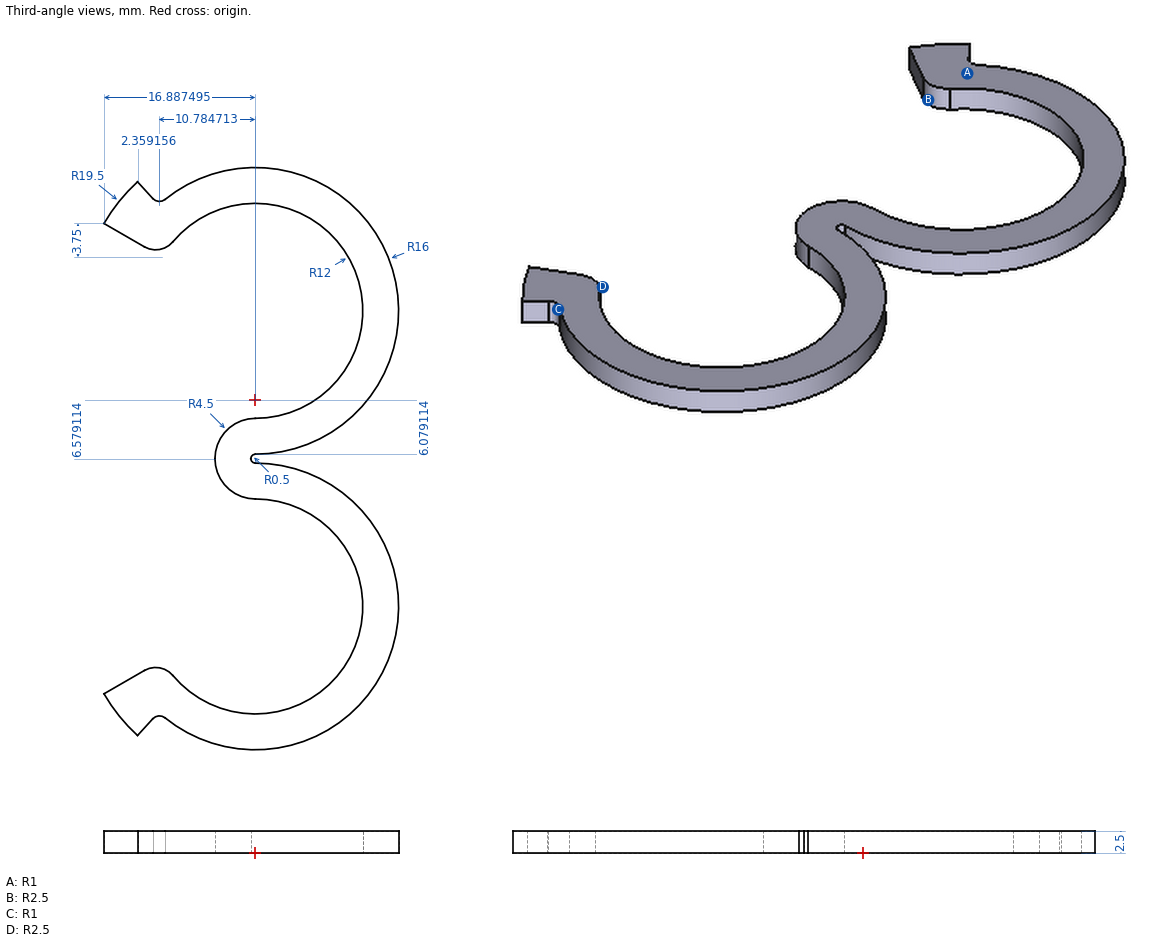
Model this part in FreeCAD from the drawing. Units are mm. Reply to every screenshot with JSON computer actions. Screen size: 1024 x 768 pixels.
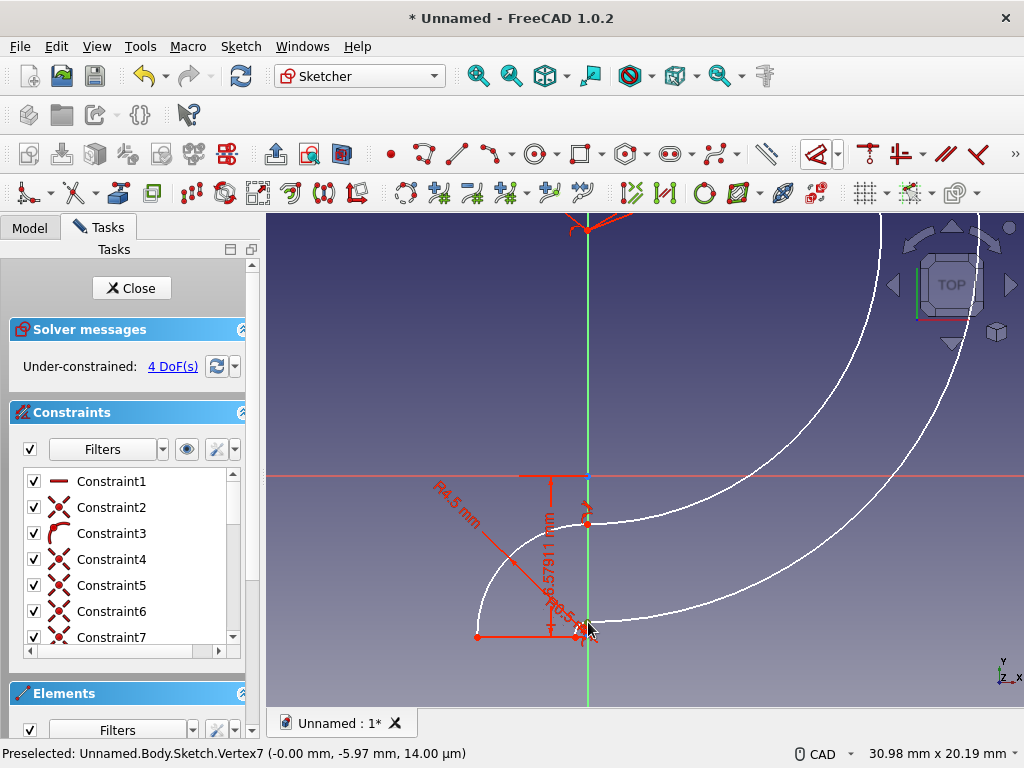
{"action": "left_click", "coordinate": [838, 154]}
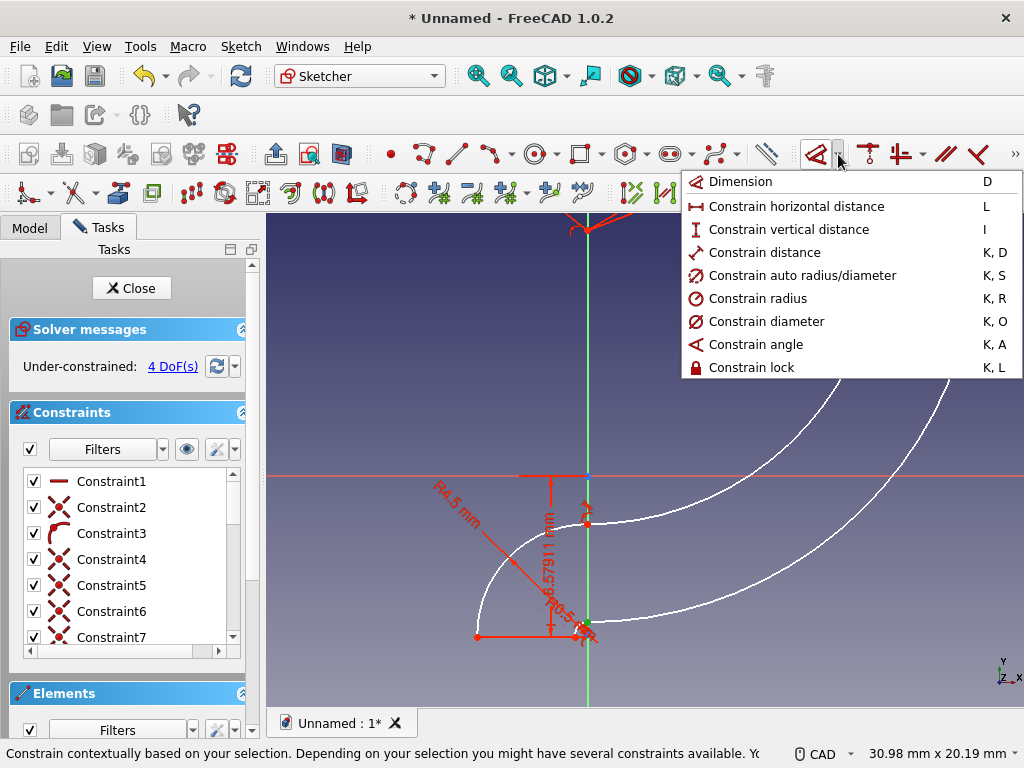
{"action": "left_click", "coordinate": [852, 230]}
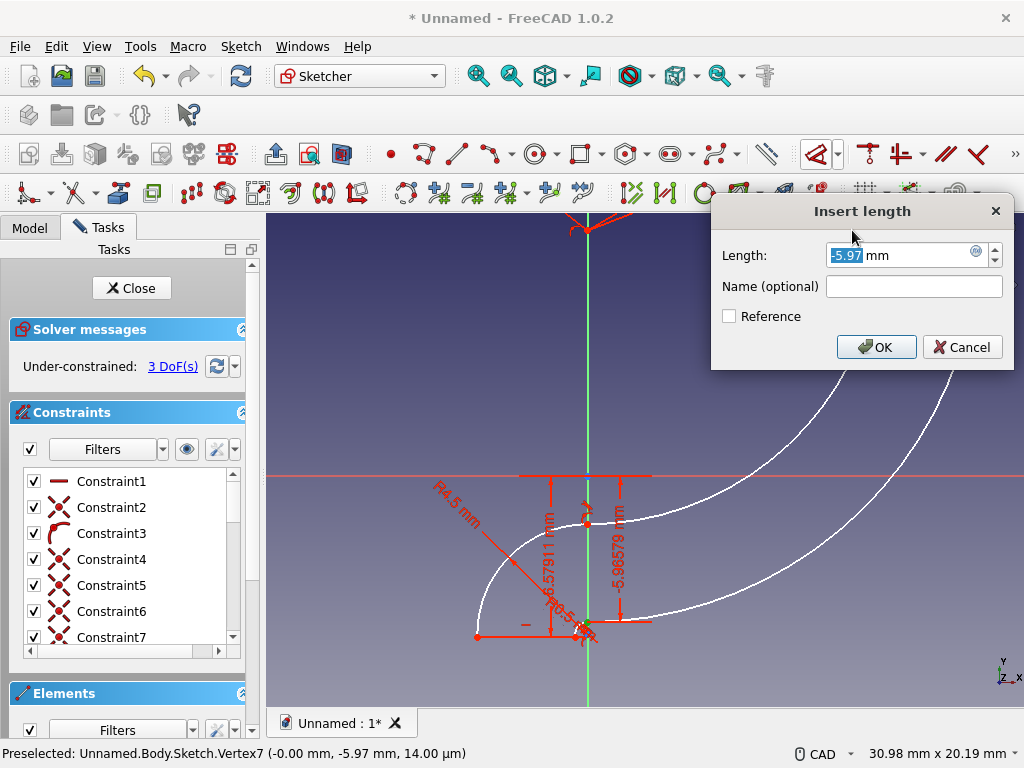
{"action": "type", "text": "-6.079114"}
{"action": "key", "text": "Return"}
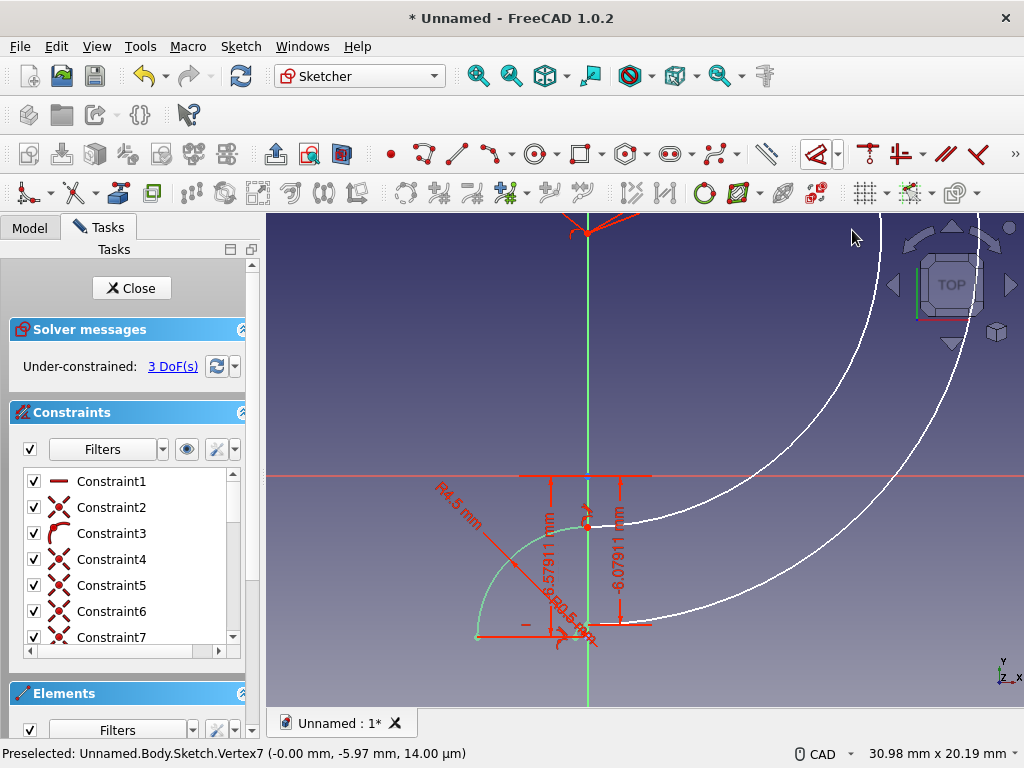
{"action": "scroll", "coordinate": [587, 624], "scroll_direction": "down", "scroll_amount": 4}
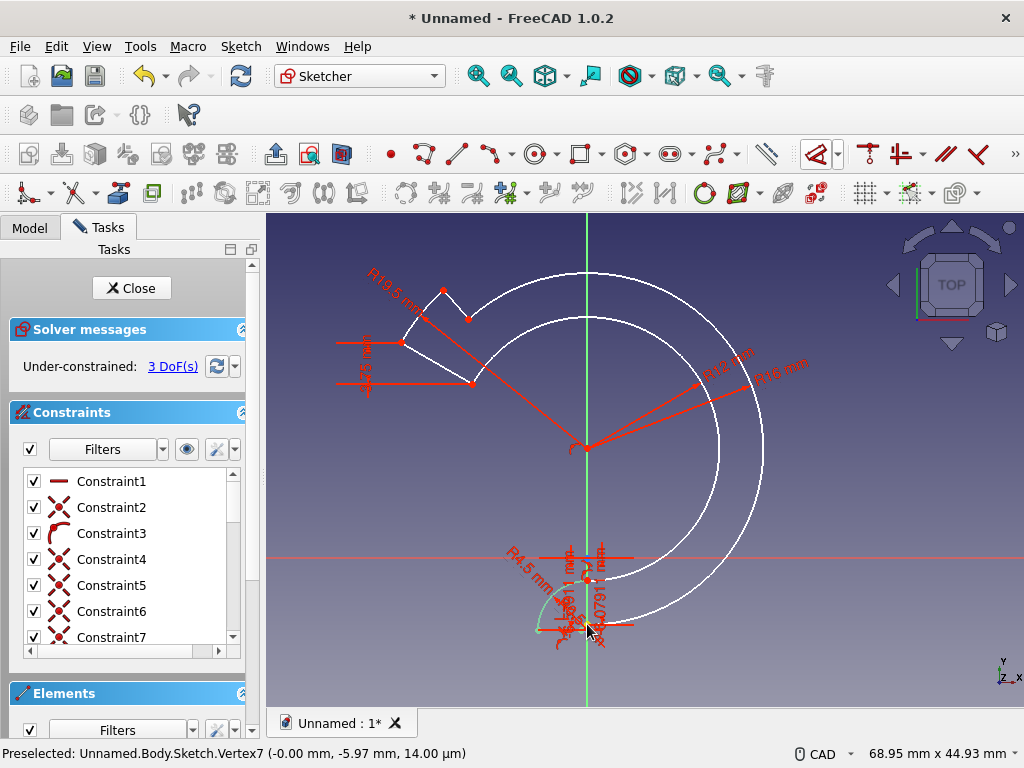
{"action": "scroll", "coordinate": [461, 310], "scroll_direction": "up", "scroll_amount": 3}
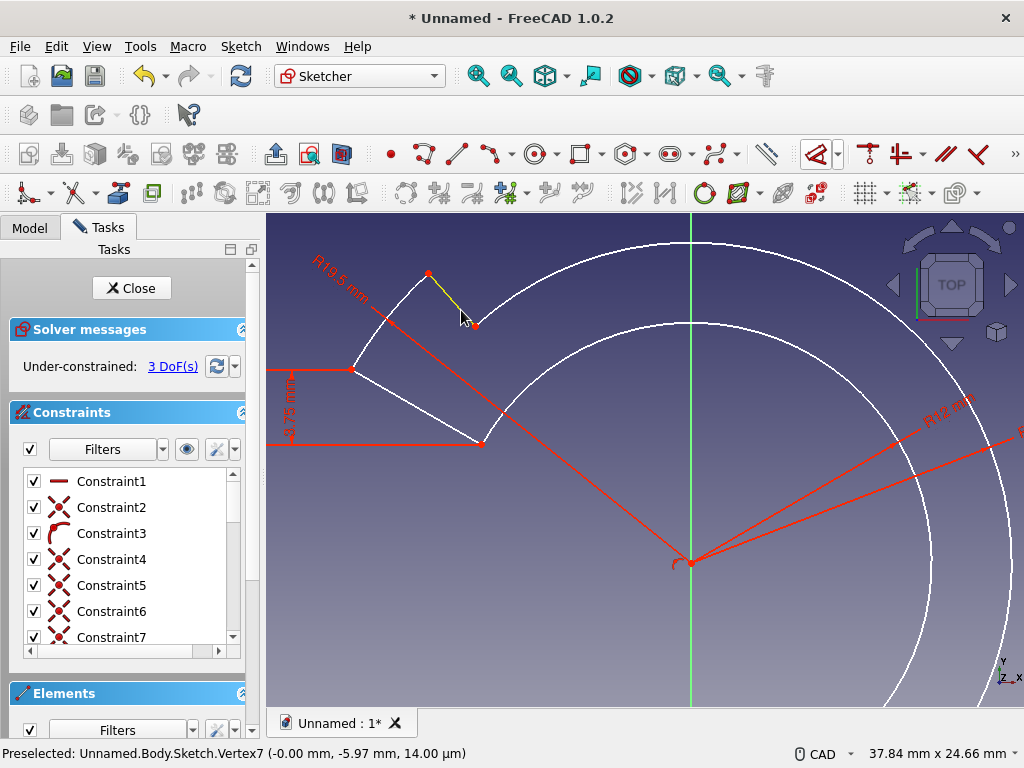
{"action": "left_click", "coordinate": [461, 311]}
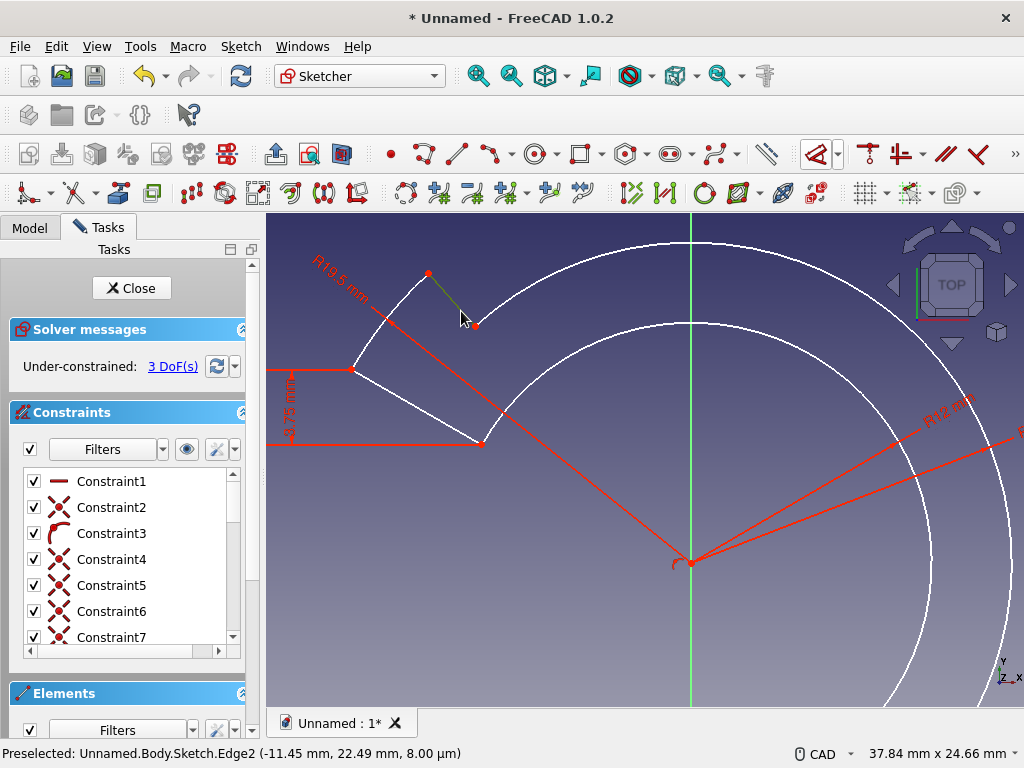
{"action": "left_click", "coordinate": [838, 154]}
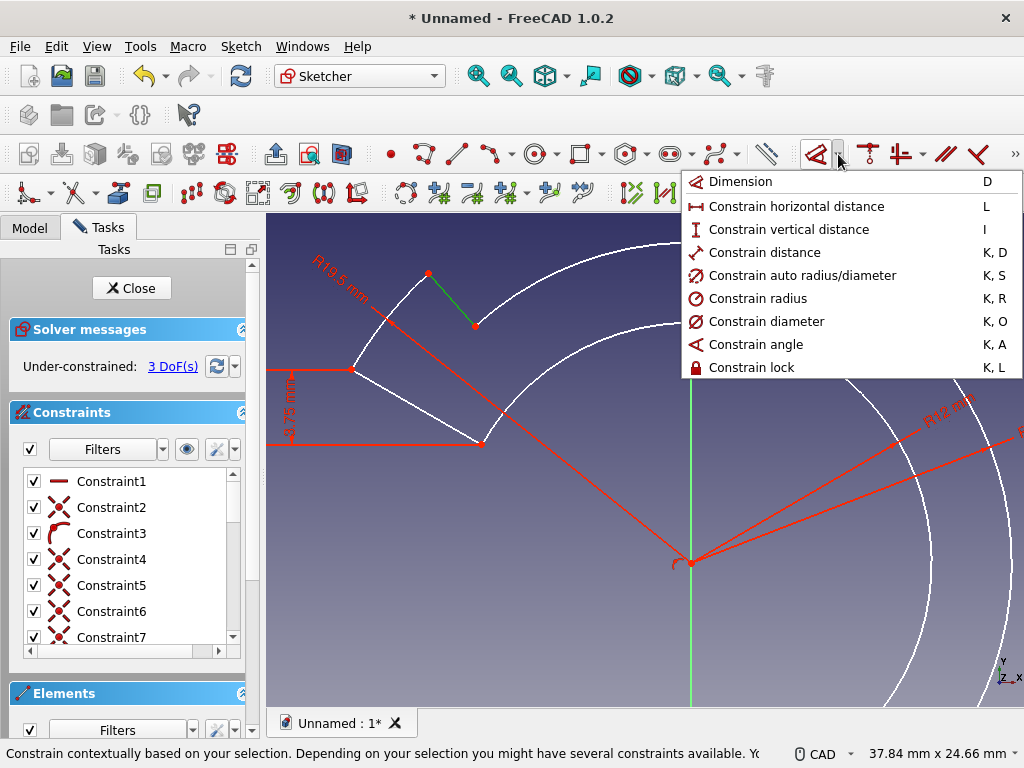
{"action": "left_click", "coordinate": [852, 206]}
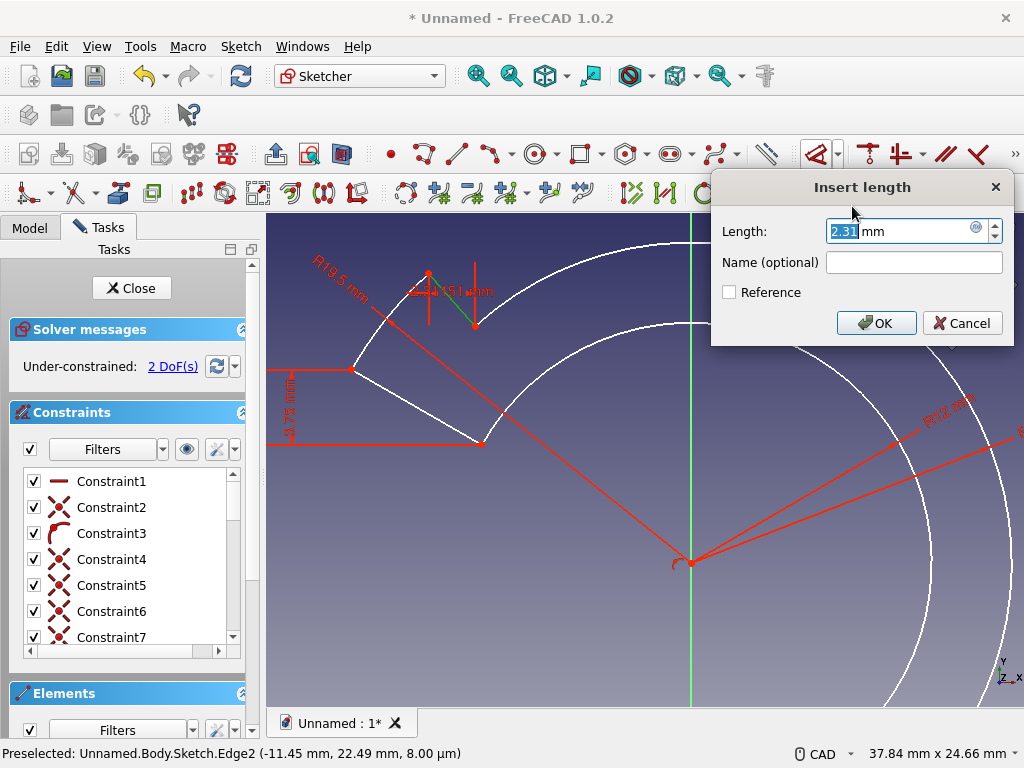
{"action": "type", "text": "2.359156"}
{"action": "key", "text": "Return"}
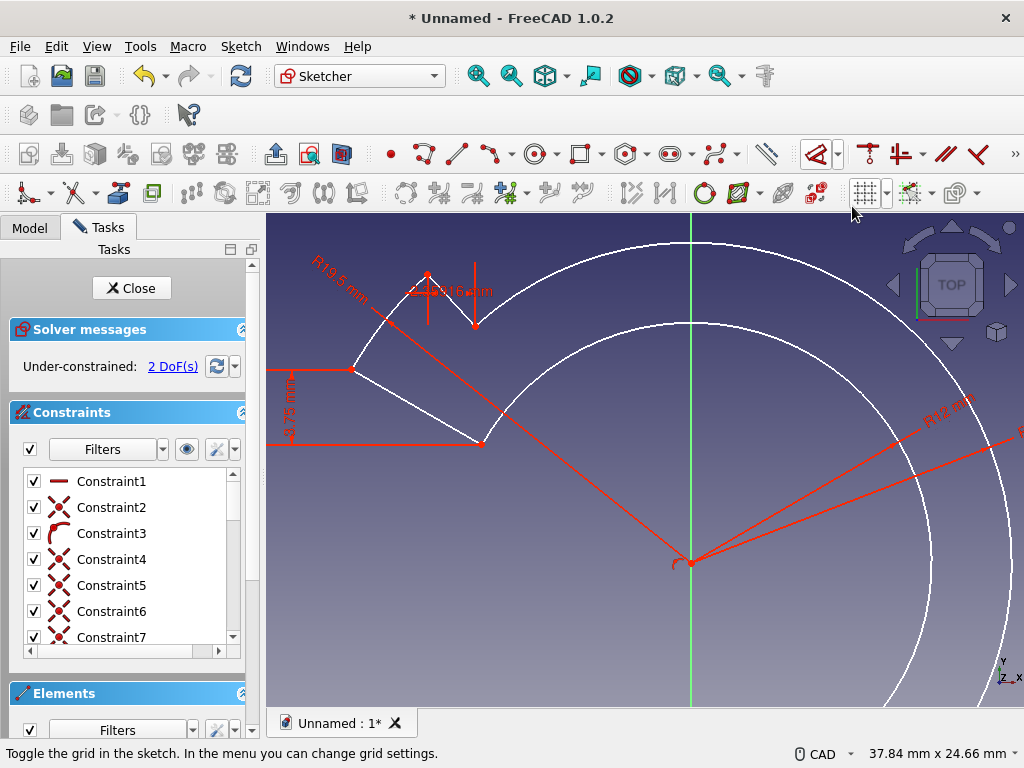
{"action": "left_click", "coordinate": [475, 326]}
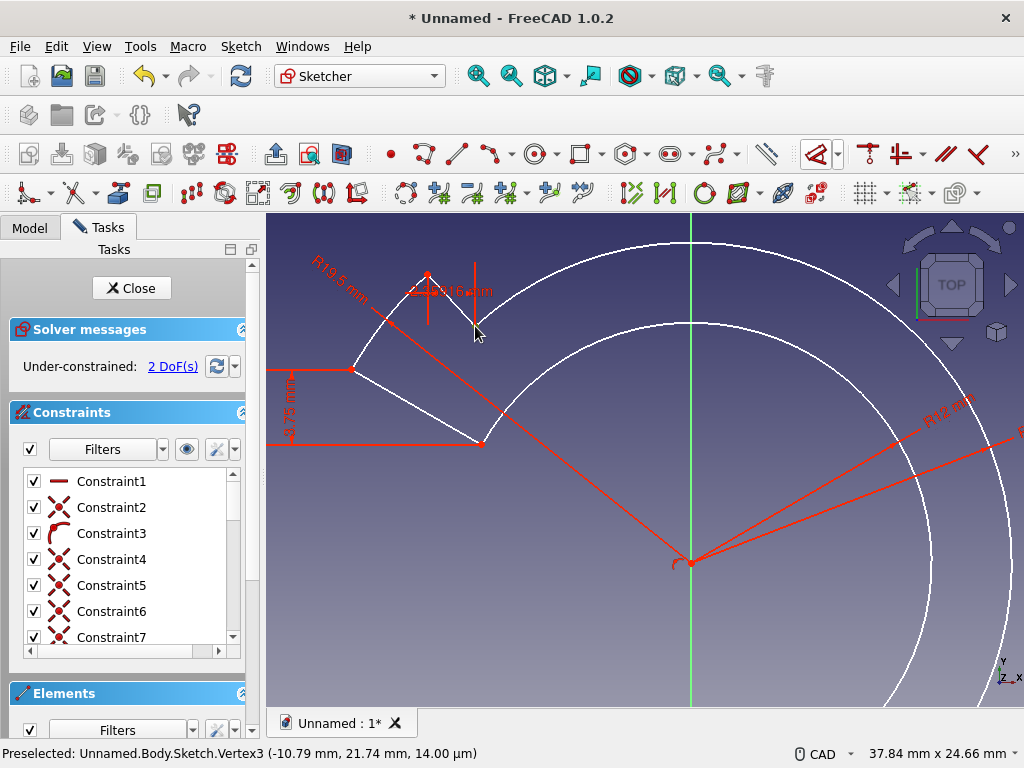
{"action": "key", "text": "l"}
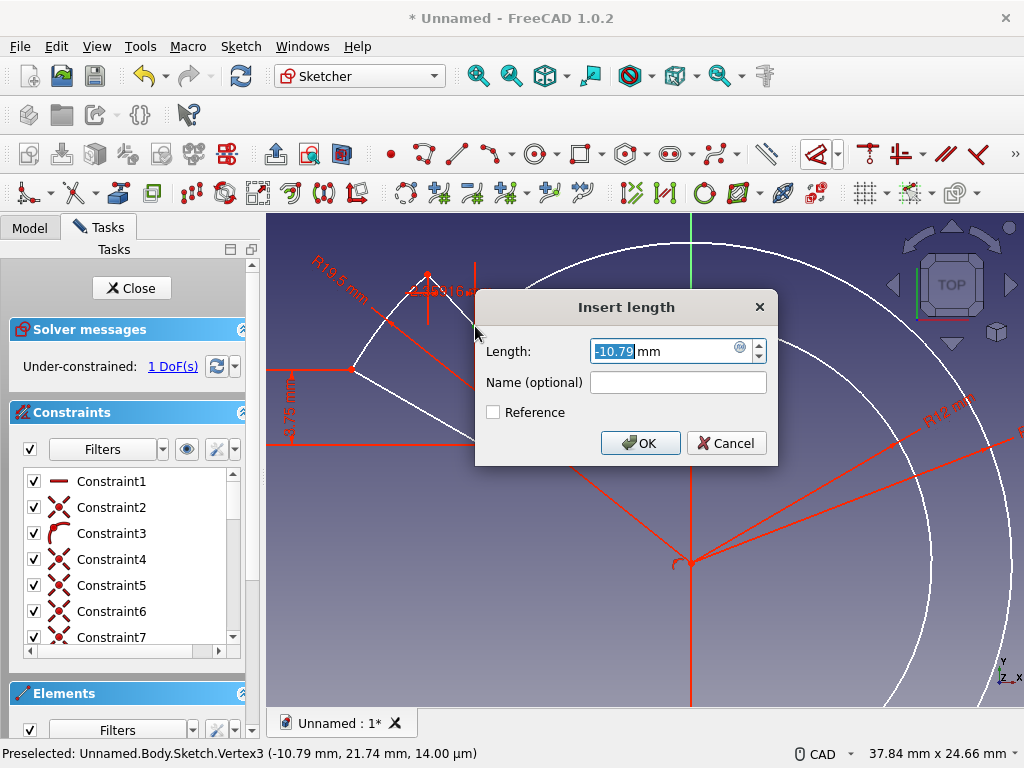
{"action": "type", "text": "-10.784713"}
{"action": "key", "text": "Return"}